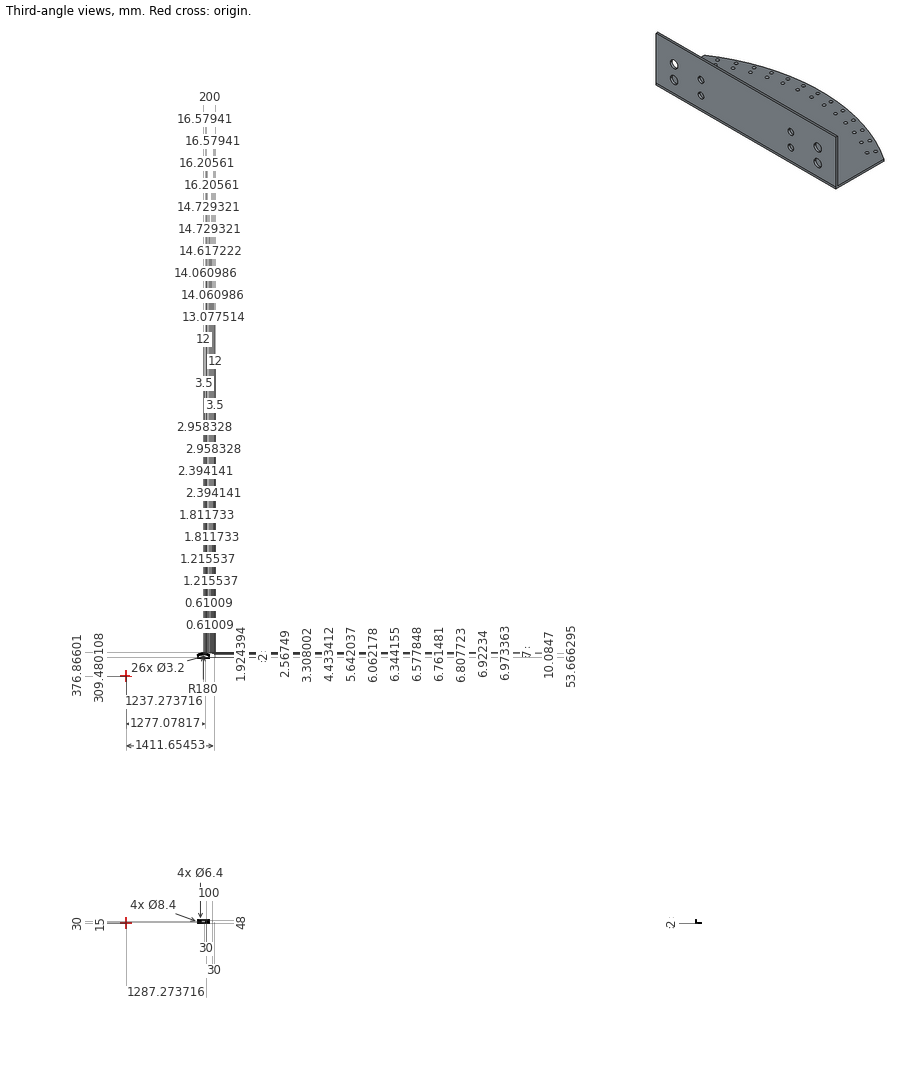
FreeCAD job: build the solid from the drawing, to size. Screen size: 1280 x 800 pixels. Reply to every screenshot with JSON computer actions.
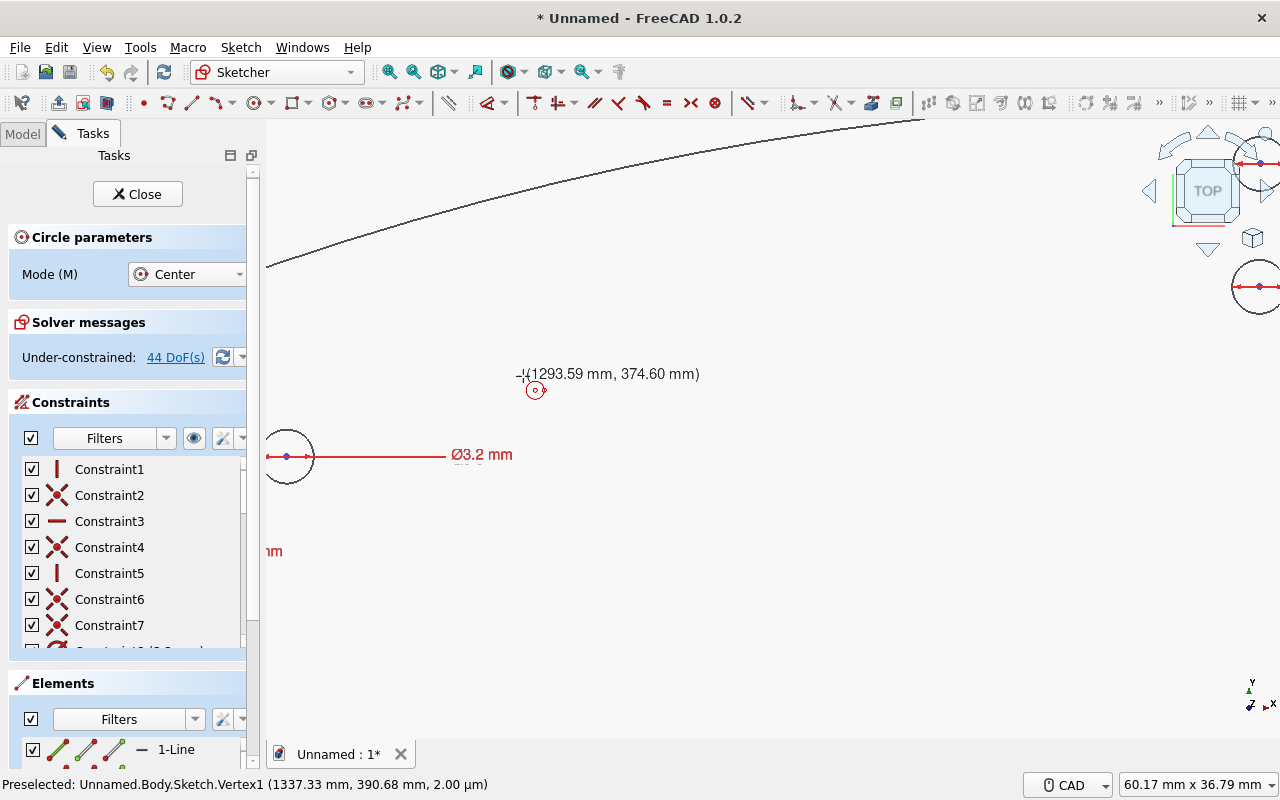
{"action": "scroll", "coordinate": [595, 355], "scroll_direction": "down", "scroll_amount": 9}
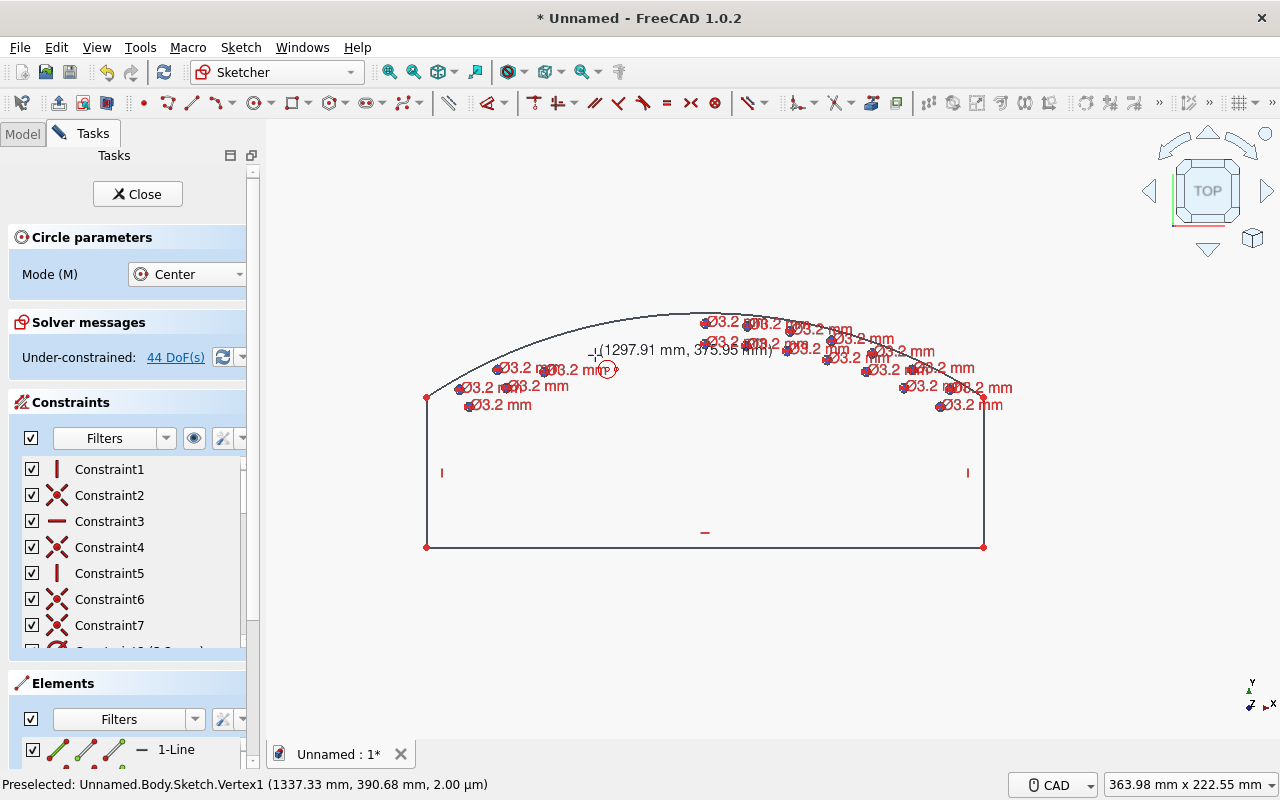
{"action": "left_click", "coordinate": [583, 359]}
{"action": "mouse_move", "coordinate": [586, 356]}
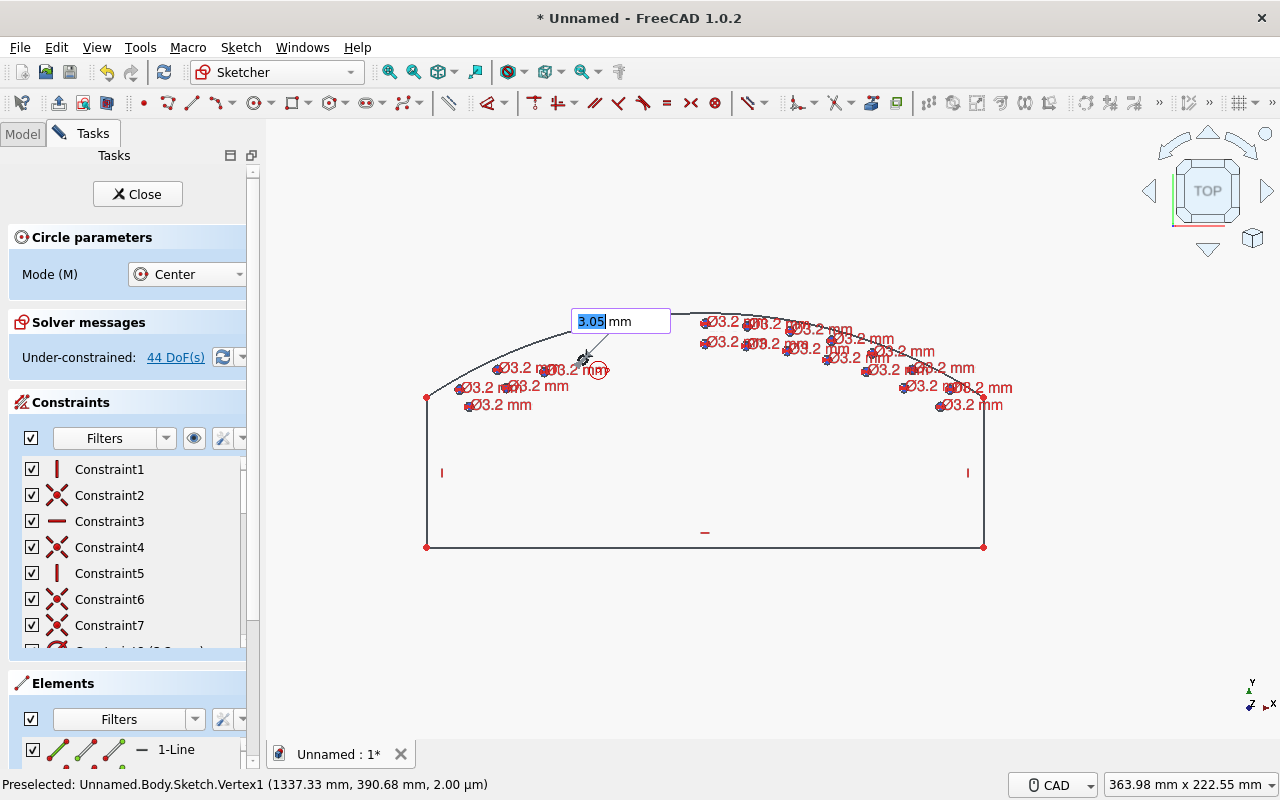
{"action": "type", "text": "3.2"}
{"action": "key", "text": "Return"}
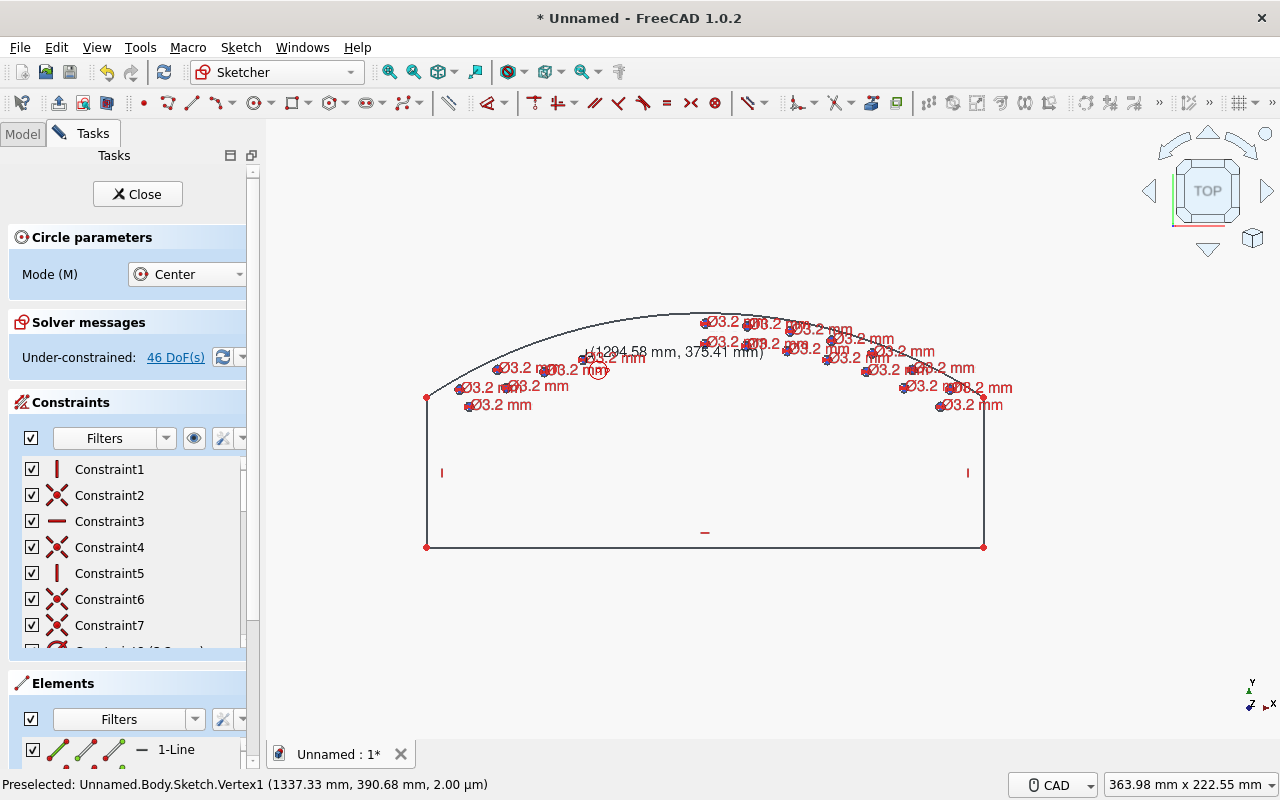
{"action": "scroll", "coordinate": [664, 345], "scroll_direction": "up", "scroll_amount": 9}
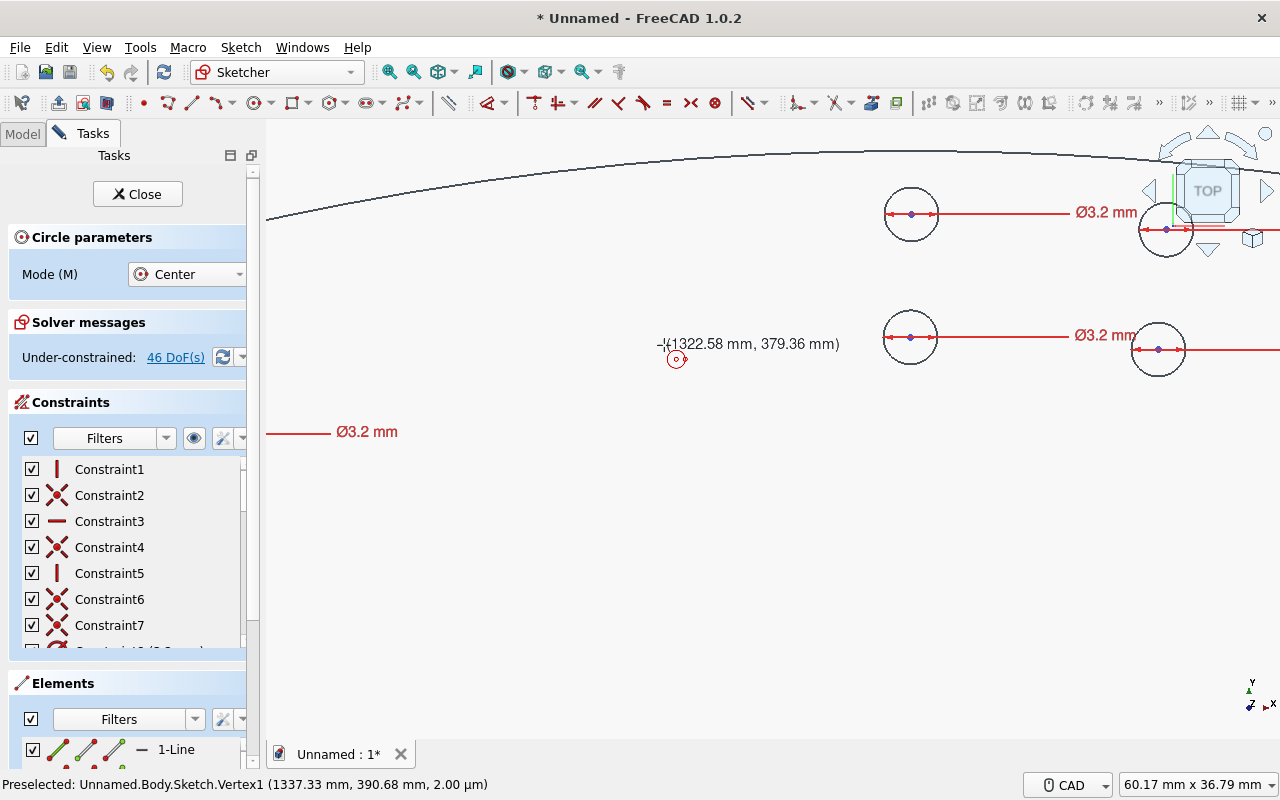
{"action": "scroll", "coordinate": [664, 345], "scroll_direction": "down", "scroll_amount": 9}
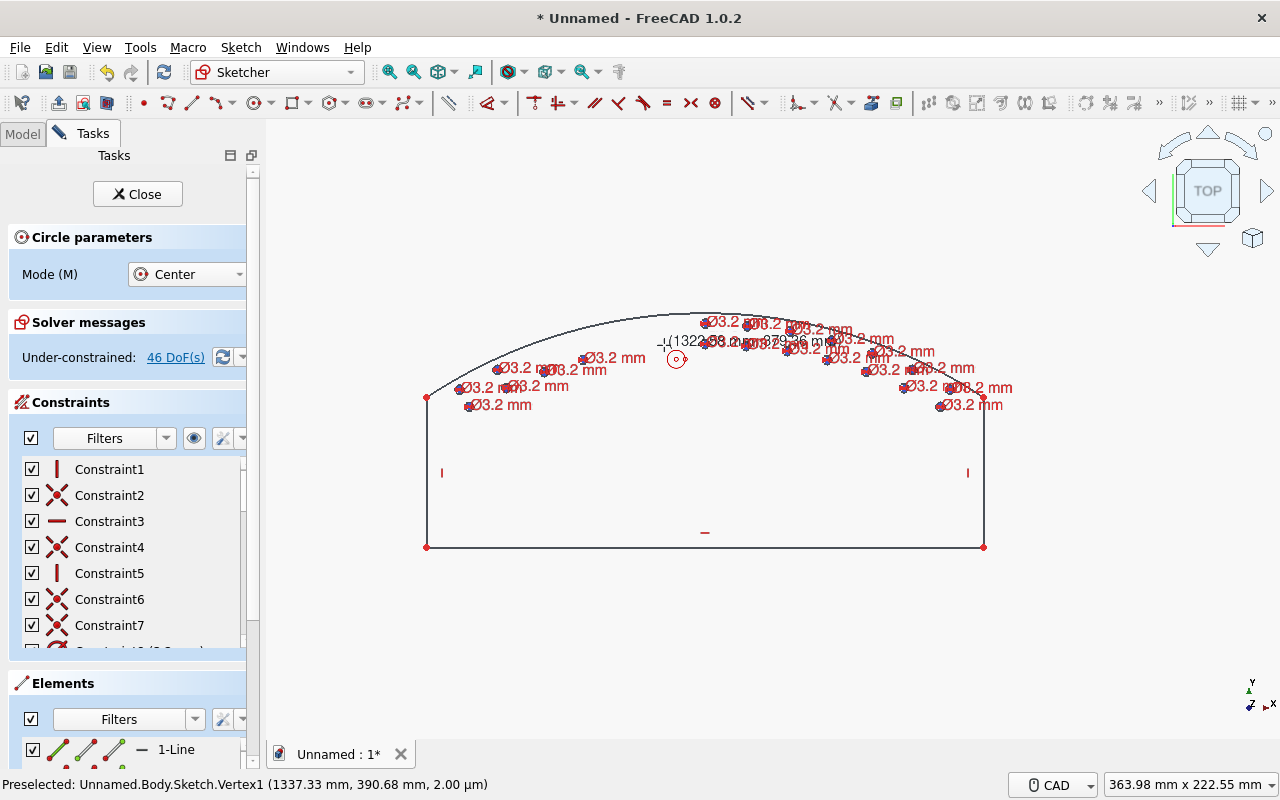
{"action": "left_click", "coordinate": [664, 345]}
{"action": "mouse_move", "coordinate": [667, 342]}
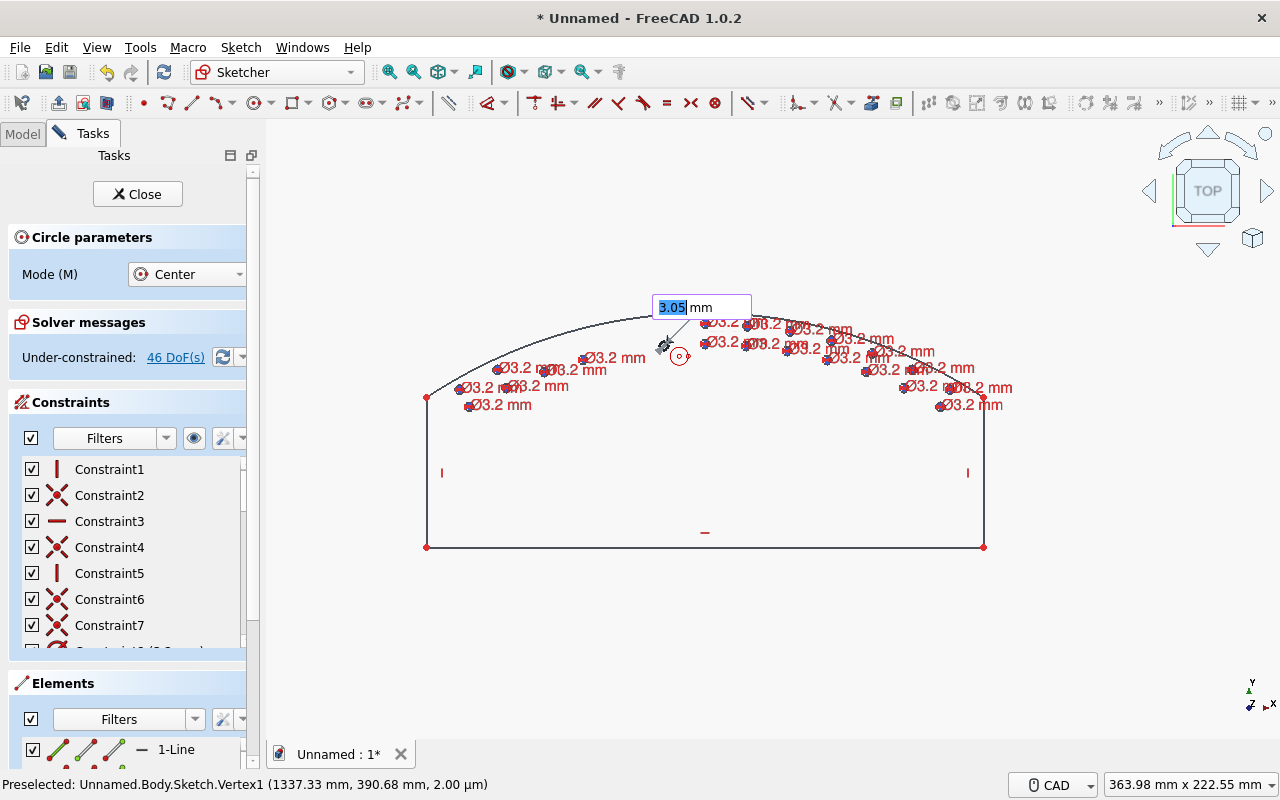
{"action": "type", "text": "3.2"}
{"action": "key", "text": "Return"}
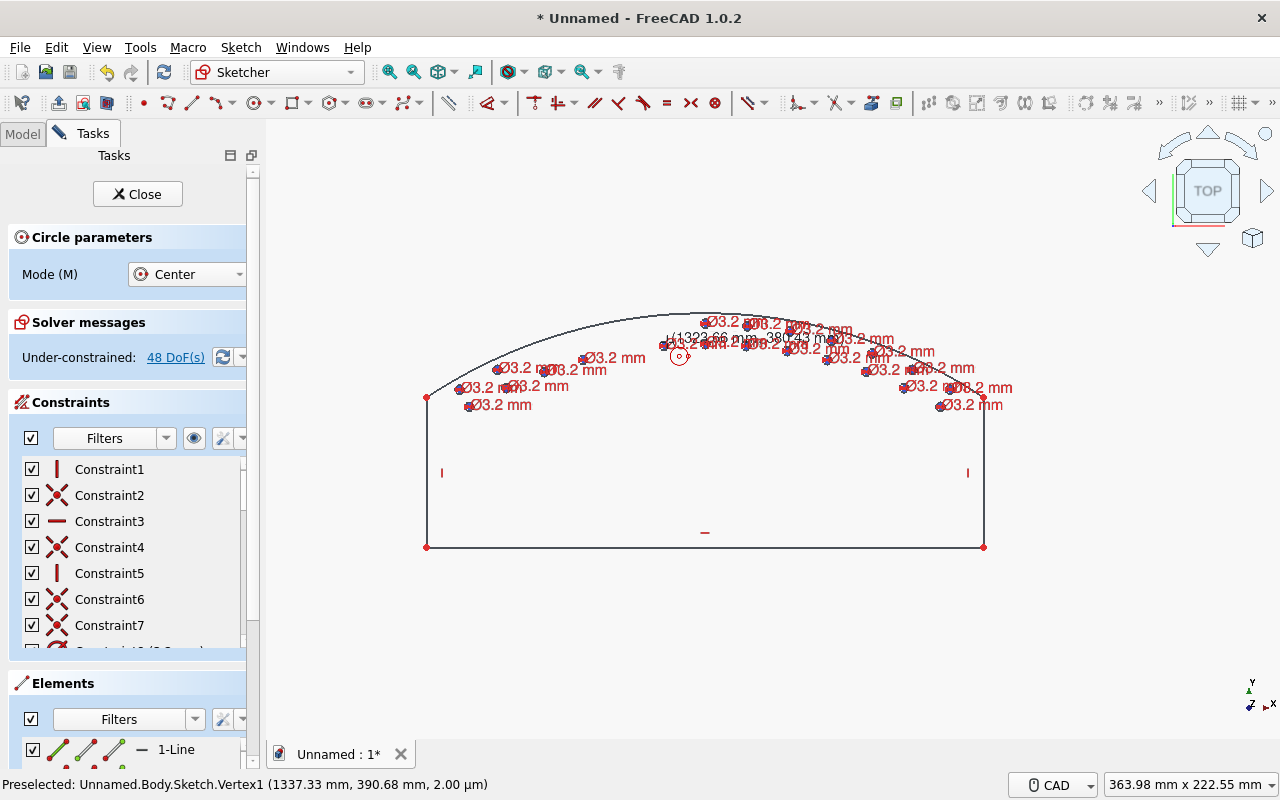
{"action": "scroll", "coordinate": [623, 350], "scroll_direction": "up", "scroll_amount": 9}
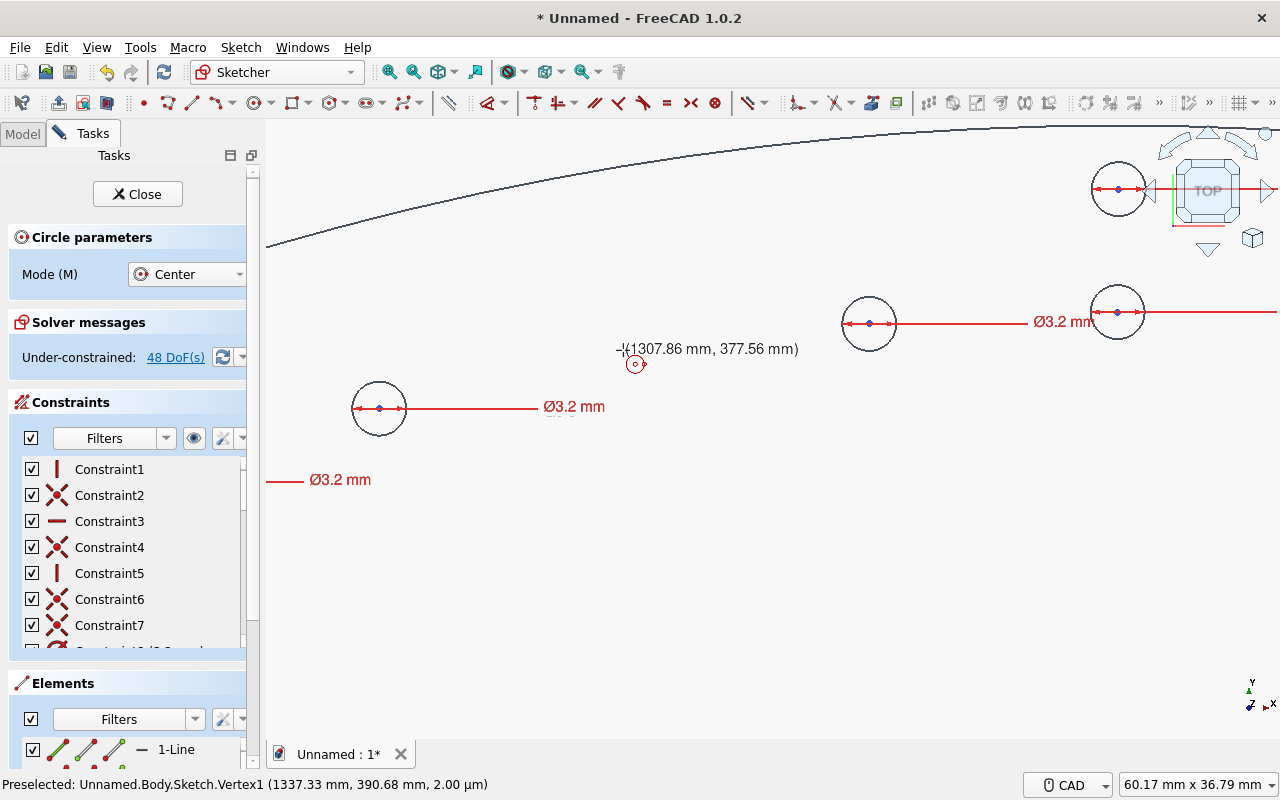
{"action": "scroll", "coordinate": [623, 350], "scroll_direction": "down", "scroll_amount": 9}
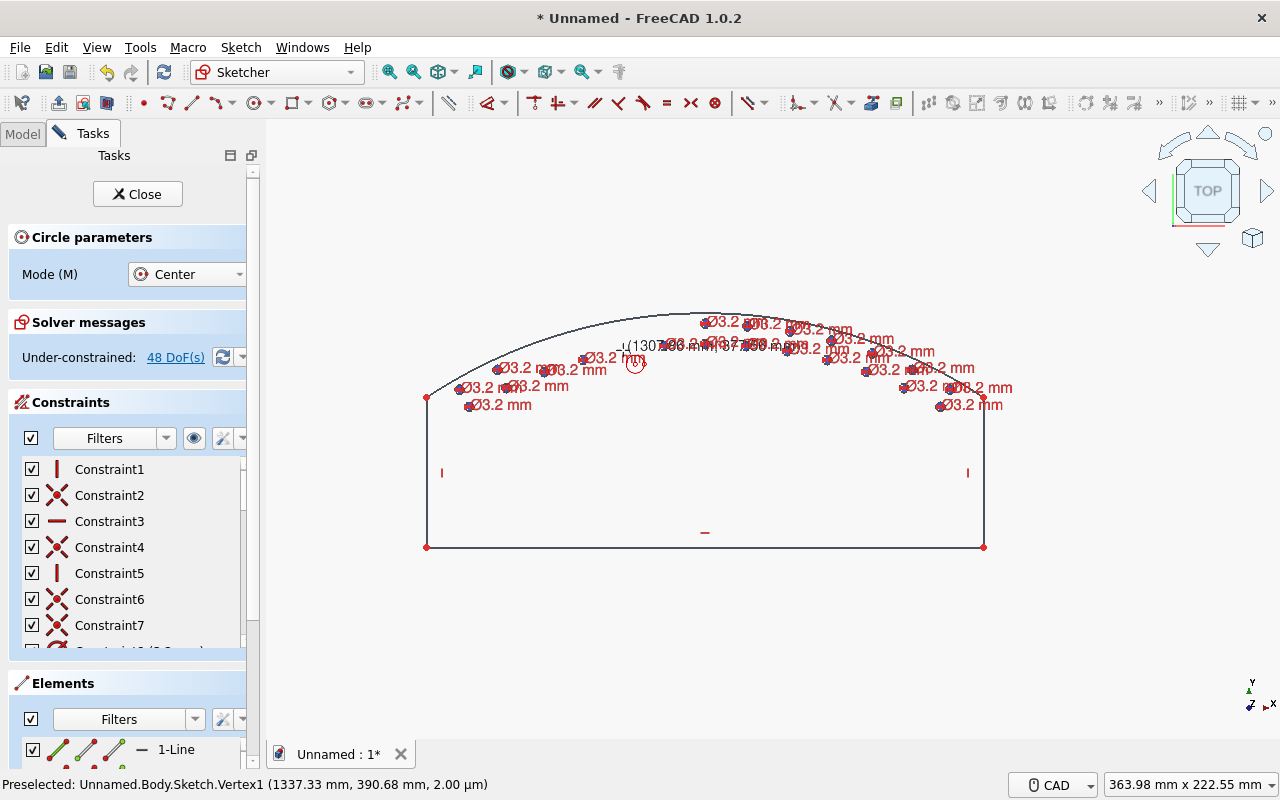
{"action": "left_click", "coordinate": [623, 350]}
{"action": "mouse_move", "coordinate": [626, 347]}